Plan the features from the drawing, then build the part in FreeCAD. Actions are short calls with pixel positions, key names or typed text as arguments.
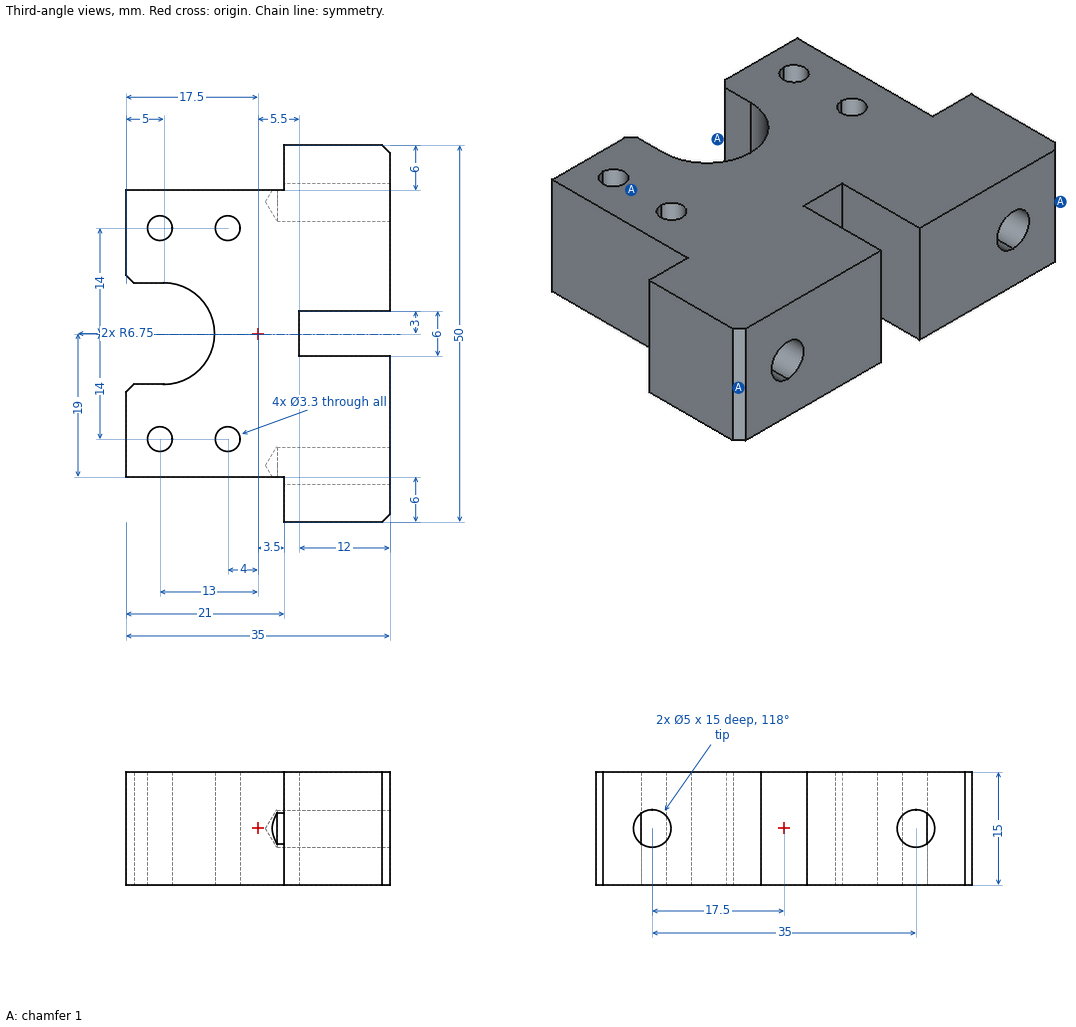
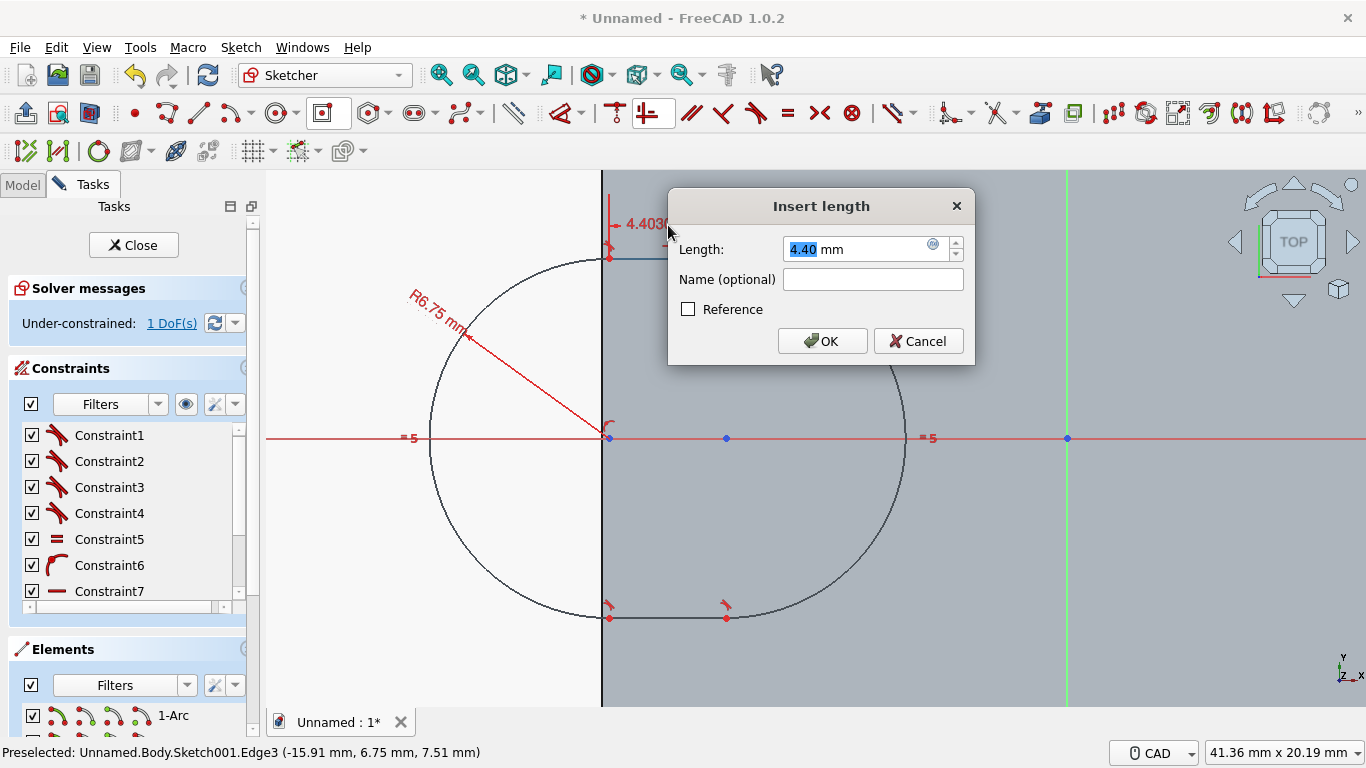
text(5)
key(Return)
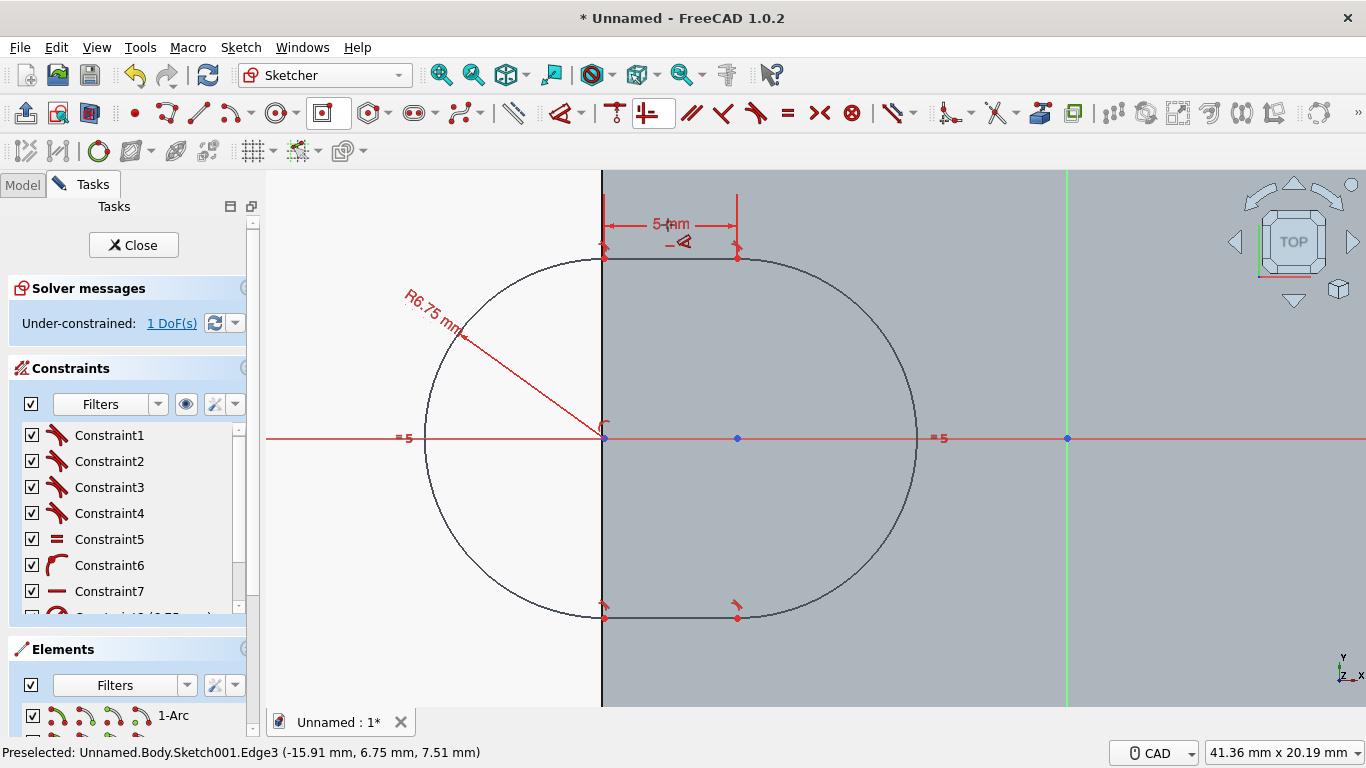
click(604, 259)
click(836, 225)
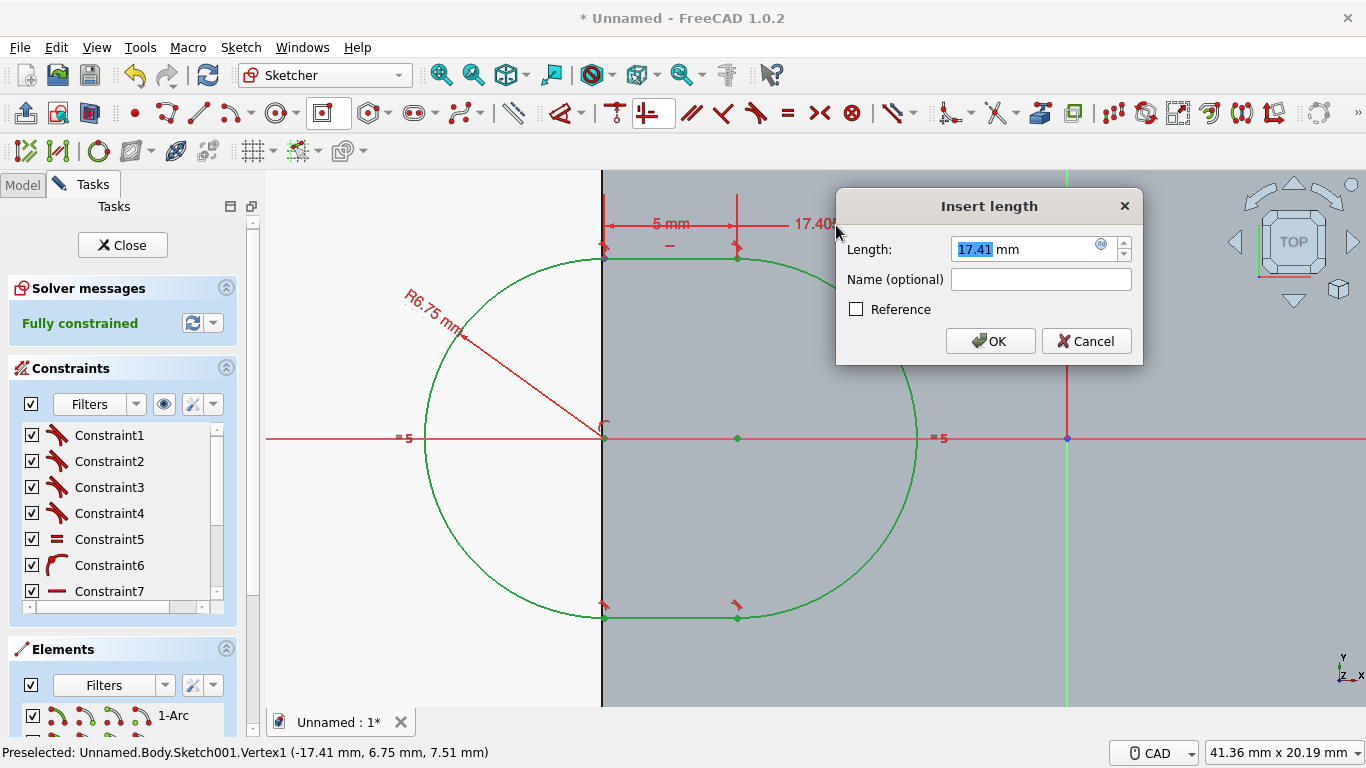
text(17.5)
key(Return)
key(Escape)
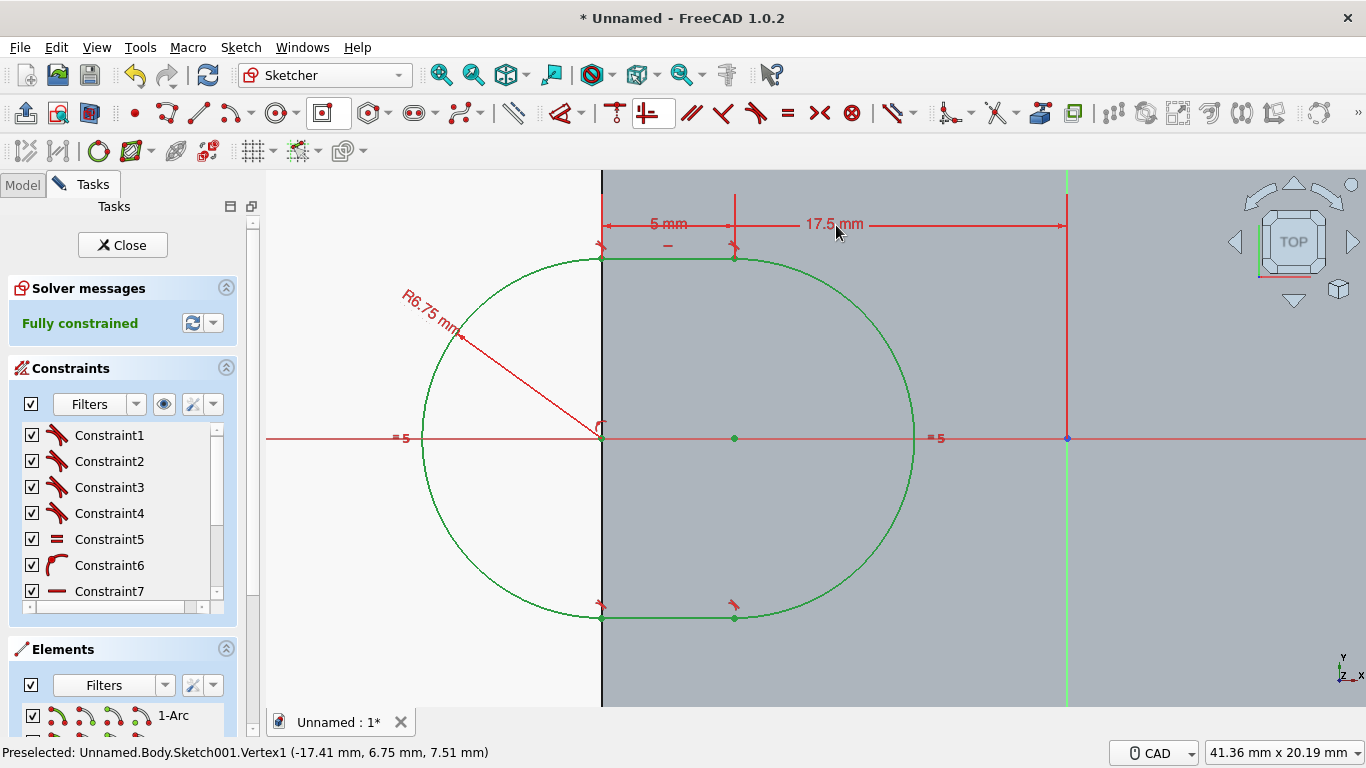
click(123, 245)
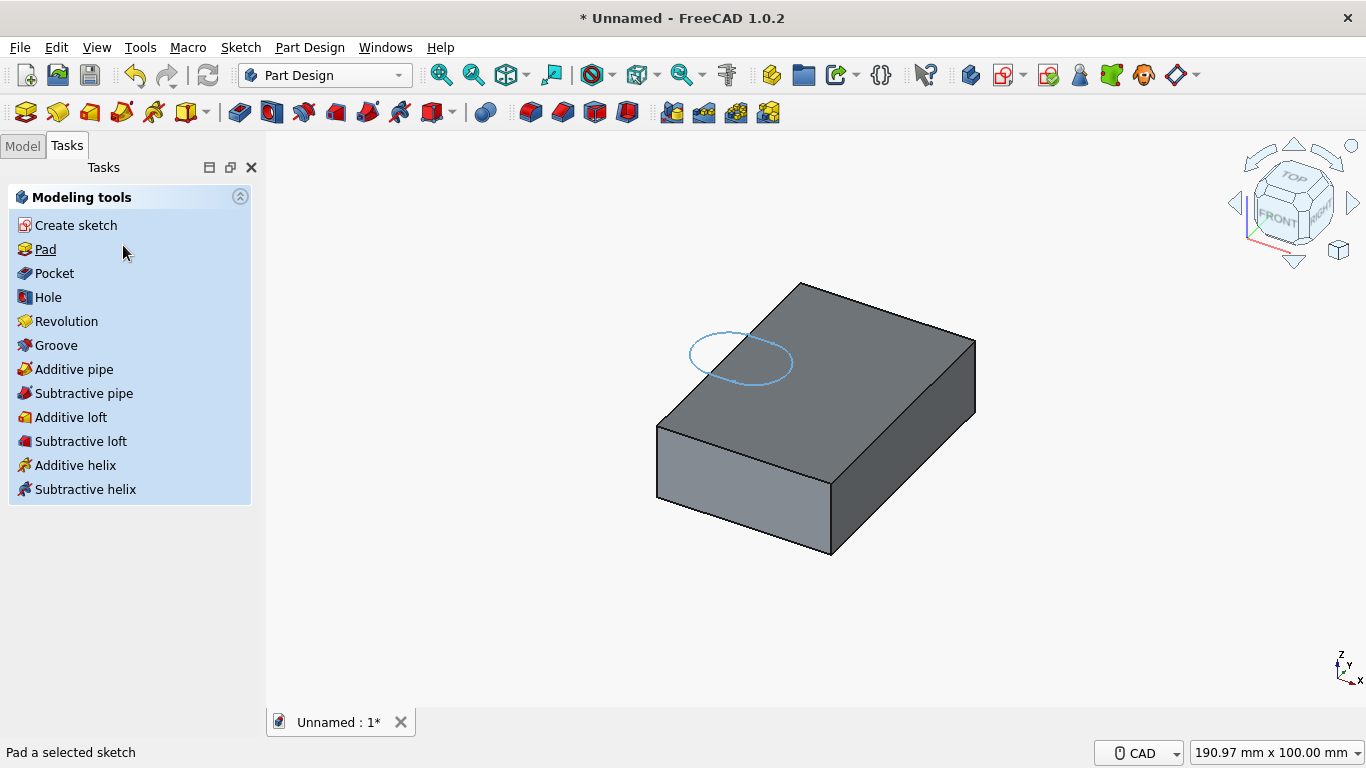
click(240, 112)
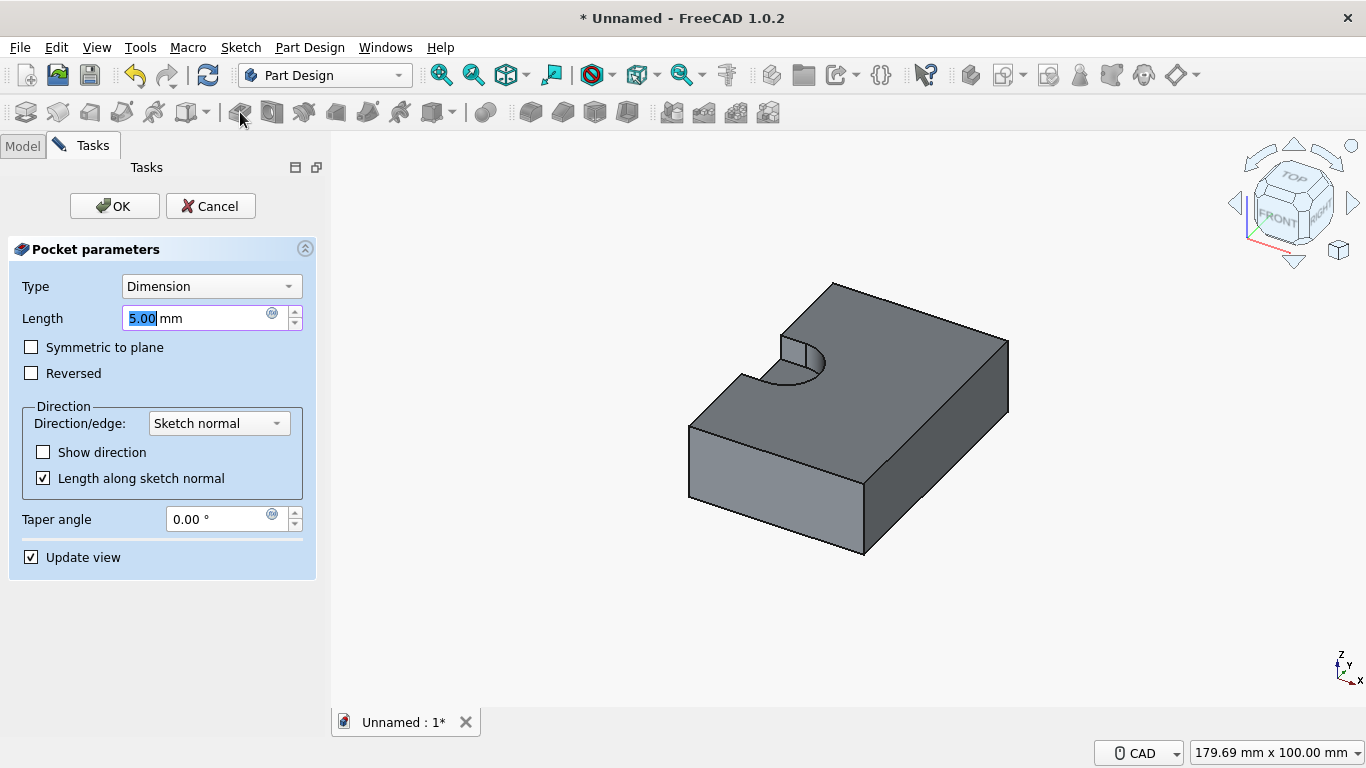
click(212, 286)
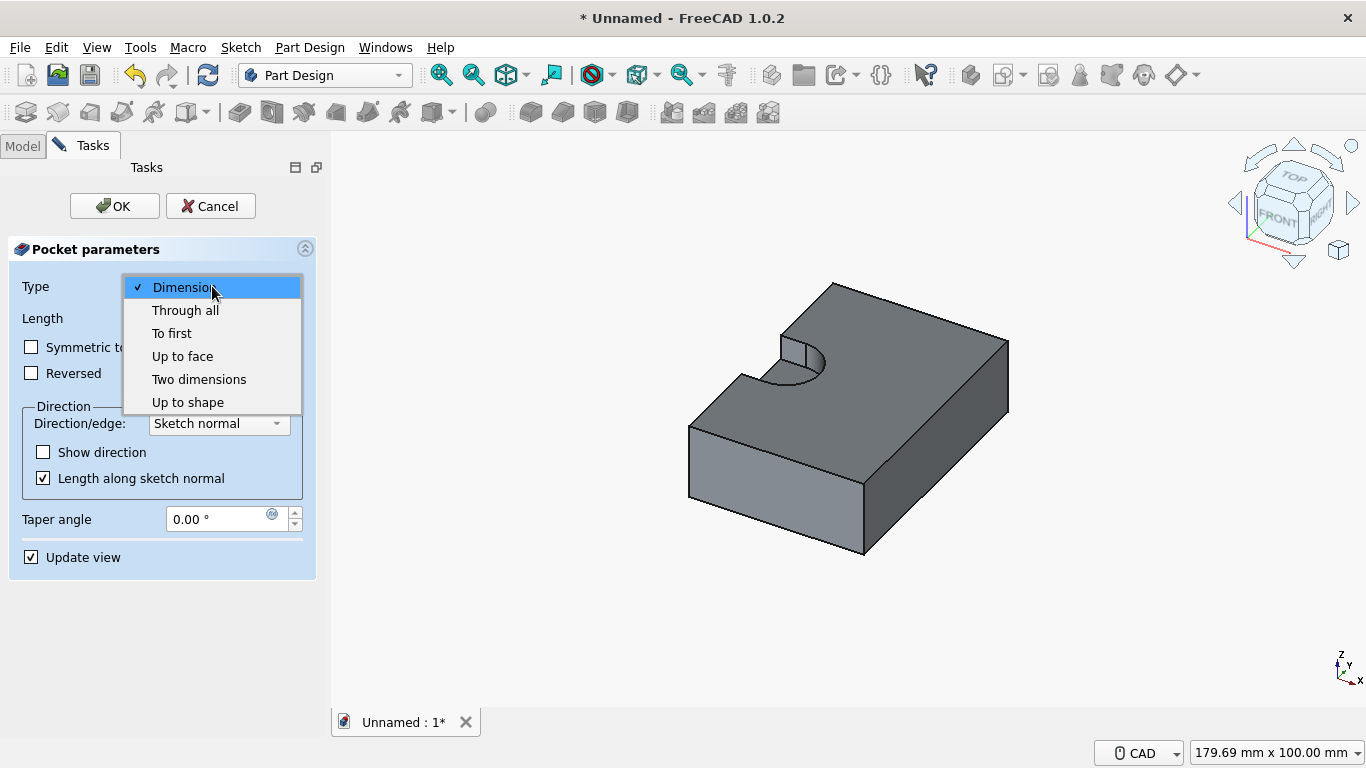
click(212, 310)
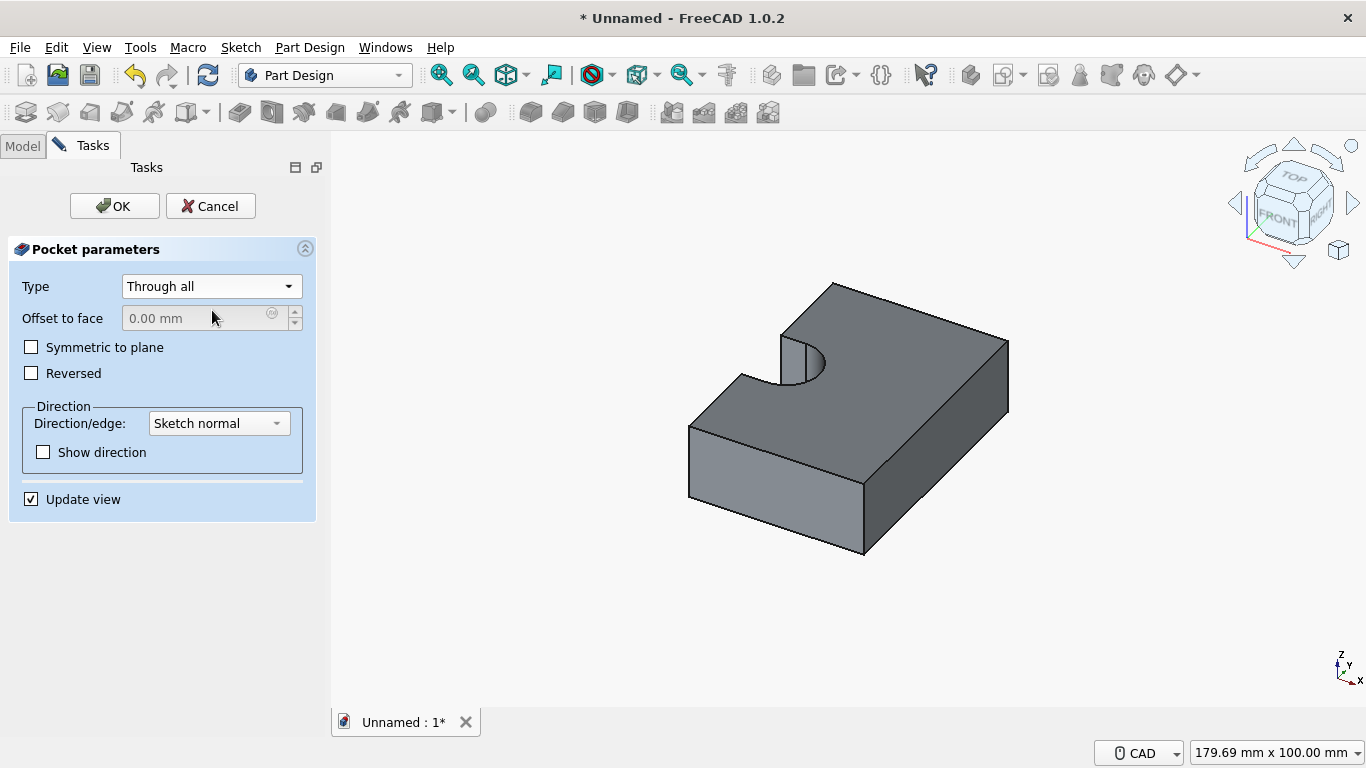
click(115, 206)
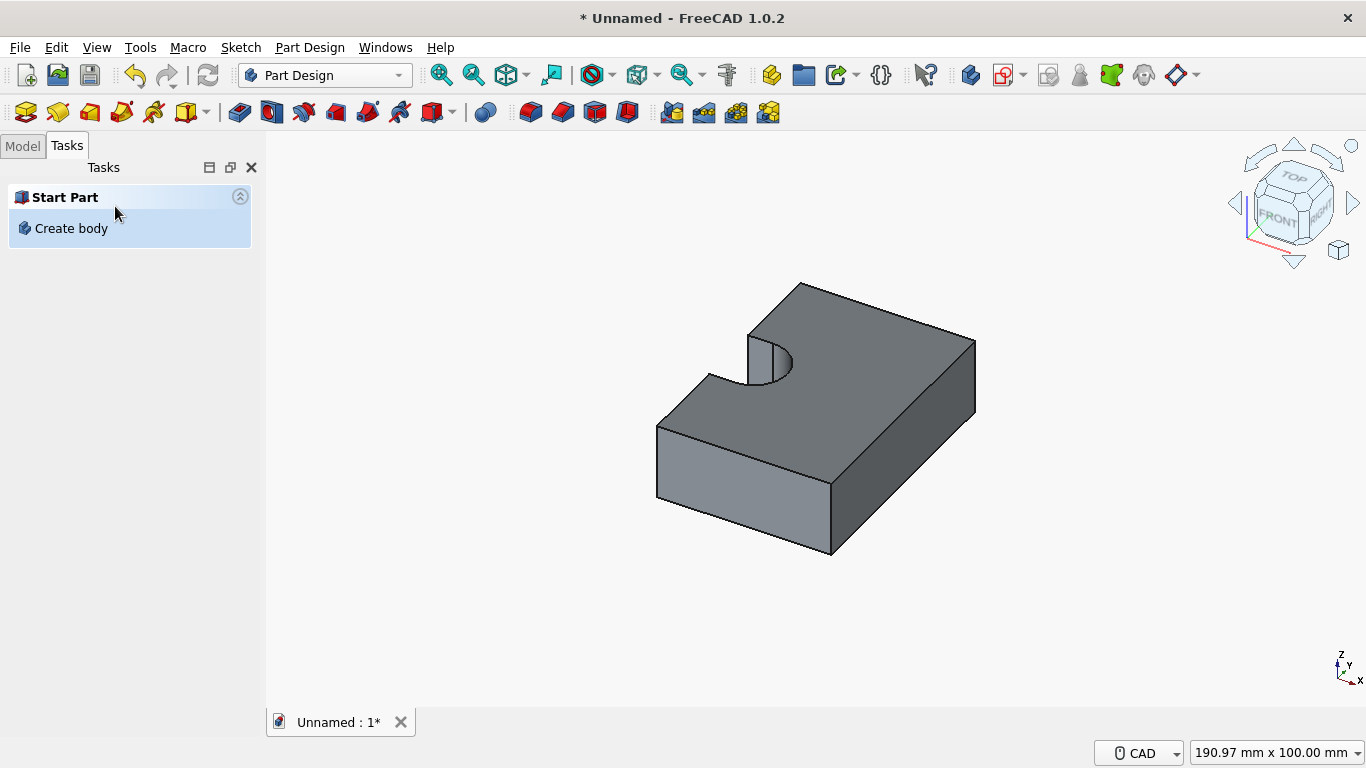
key(5)